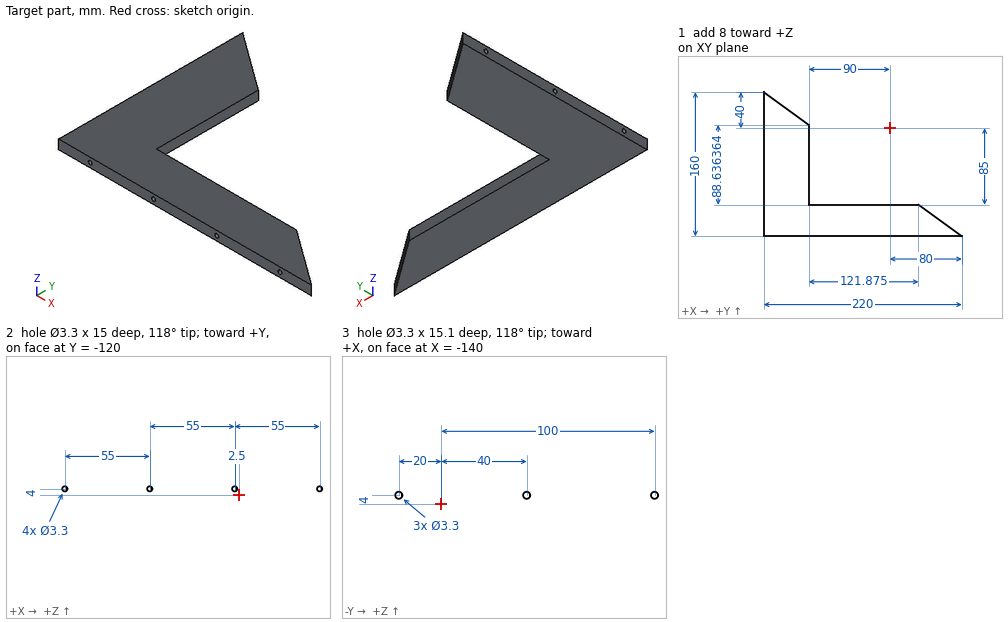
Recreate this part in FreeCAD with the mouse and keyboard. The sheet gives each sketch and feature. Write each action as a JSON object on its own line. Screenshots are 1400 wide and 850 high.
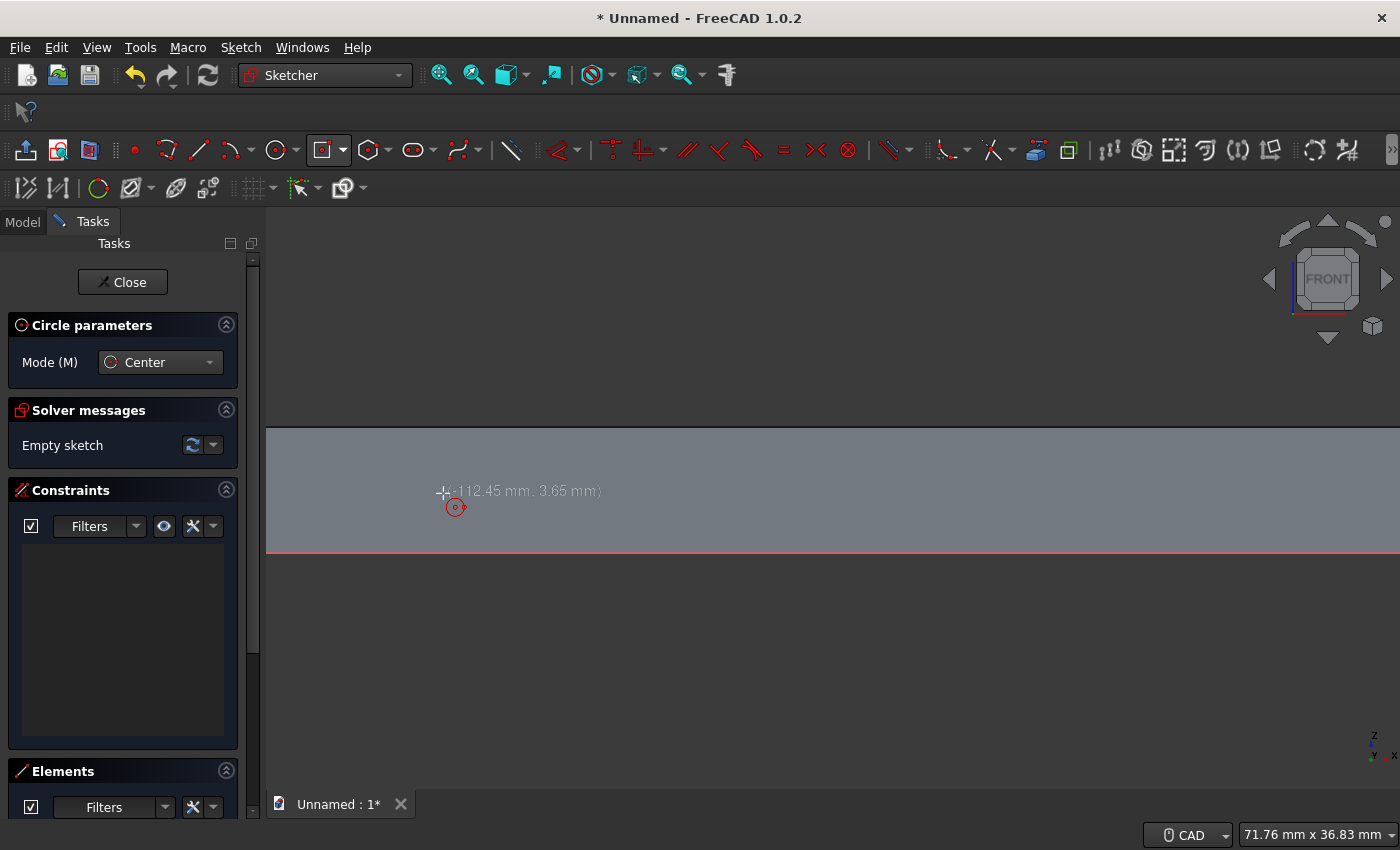
{"action": "scroll", "coordinate": [443, 495], "scroll_direction": "down", "scroll_amount": 7}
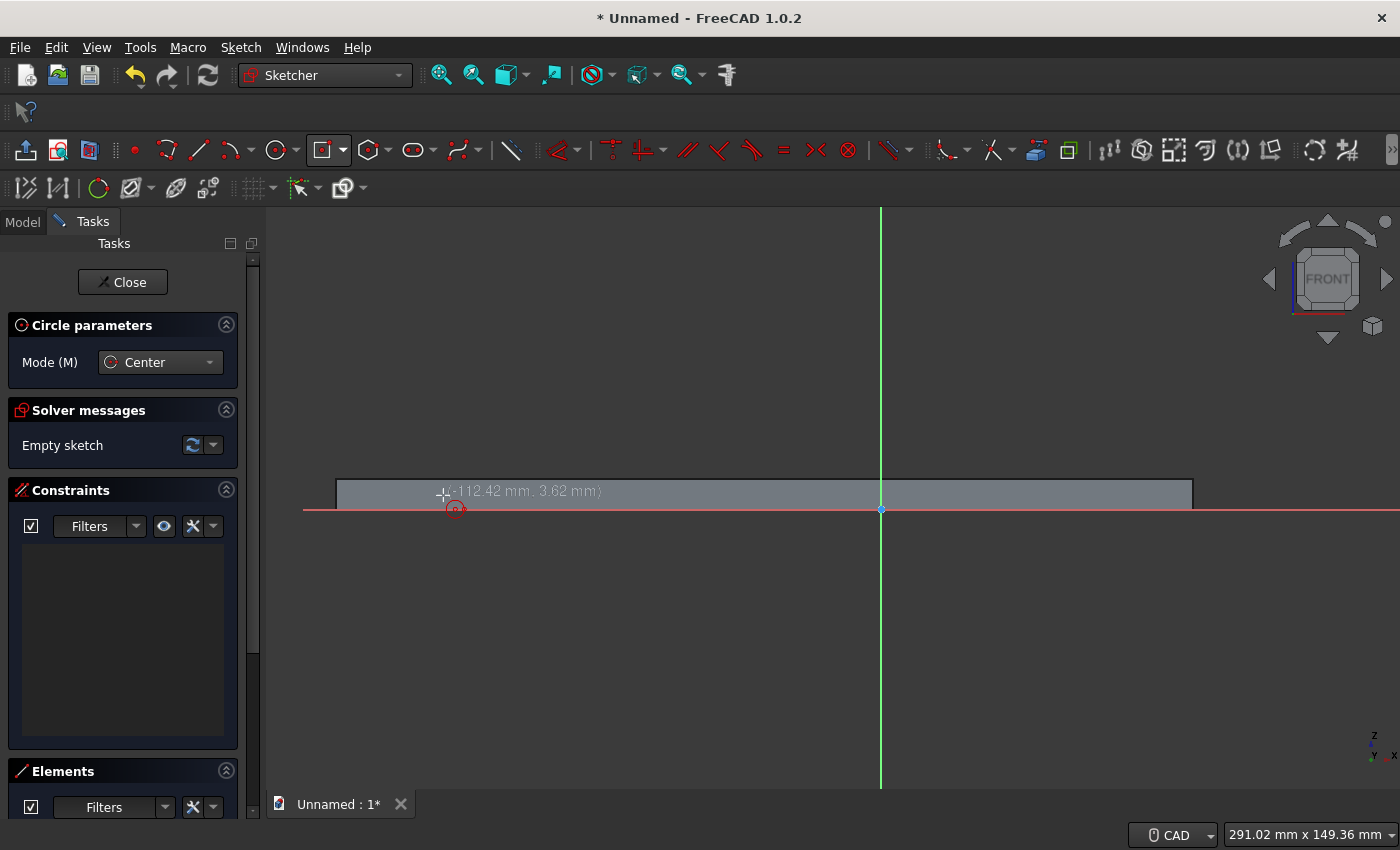
{"action": "left_click", "coordinate": [443, 494]}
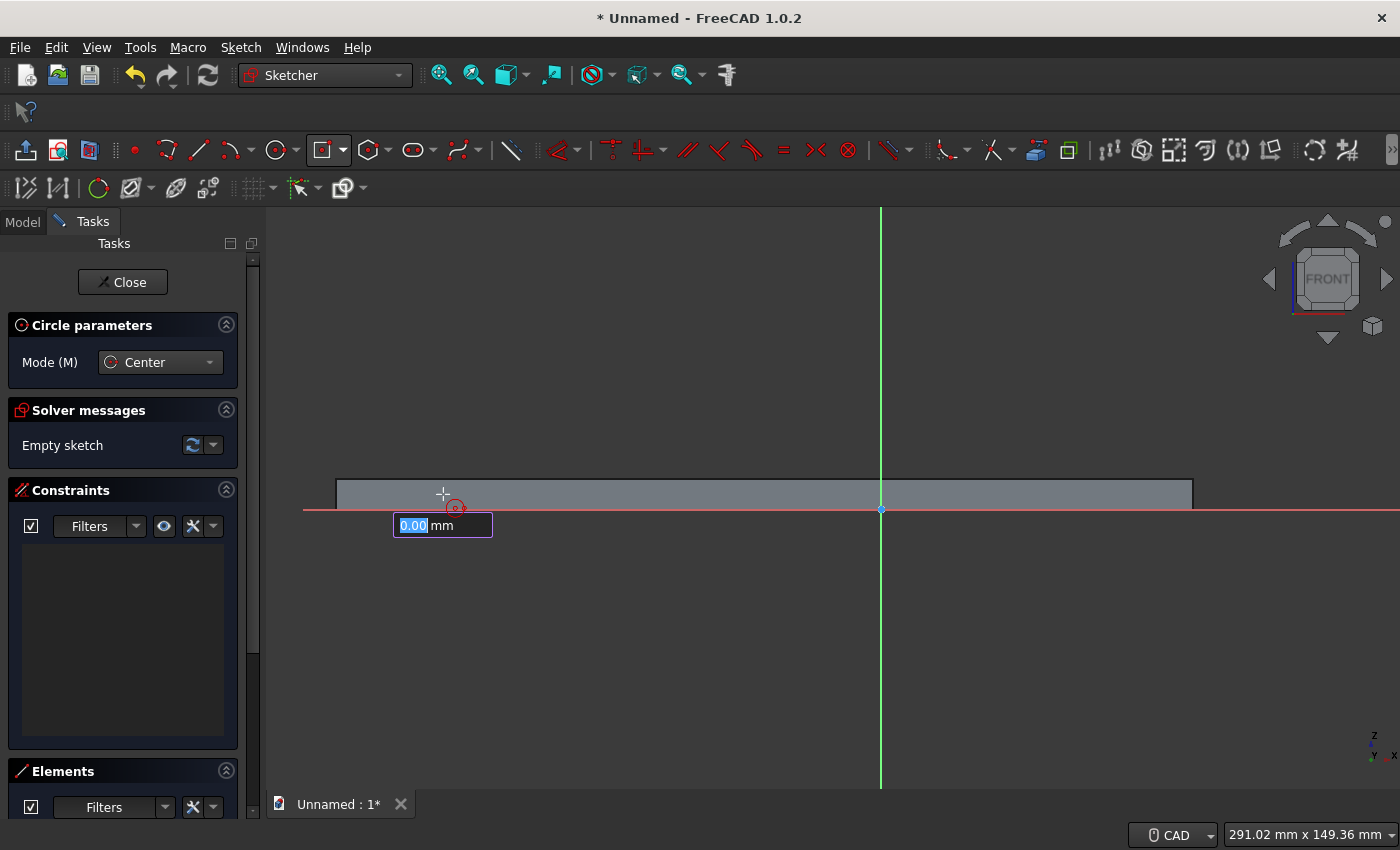
{"action": "scroll", "coordinate": [447, 490], "scroll_direction": "up", "scroll_amount": 5}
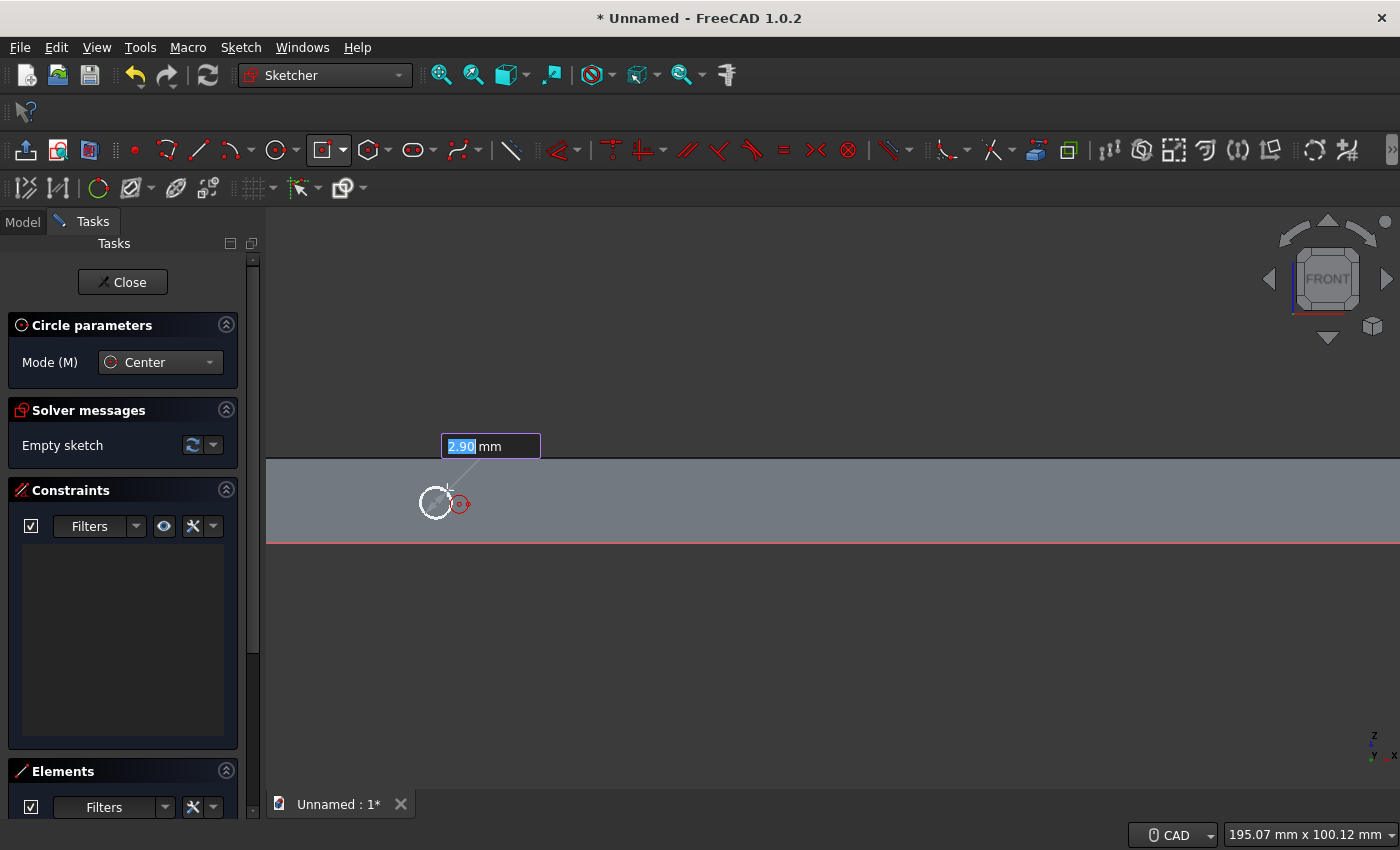
{"action": "left_click", "coordinate": [448, 488]}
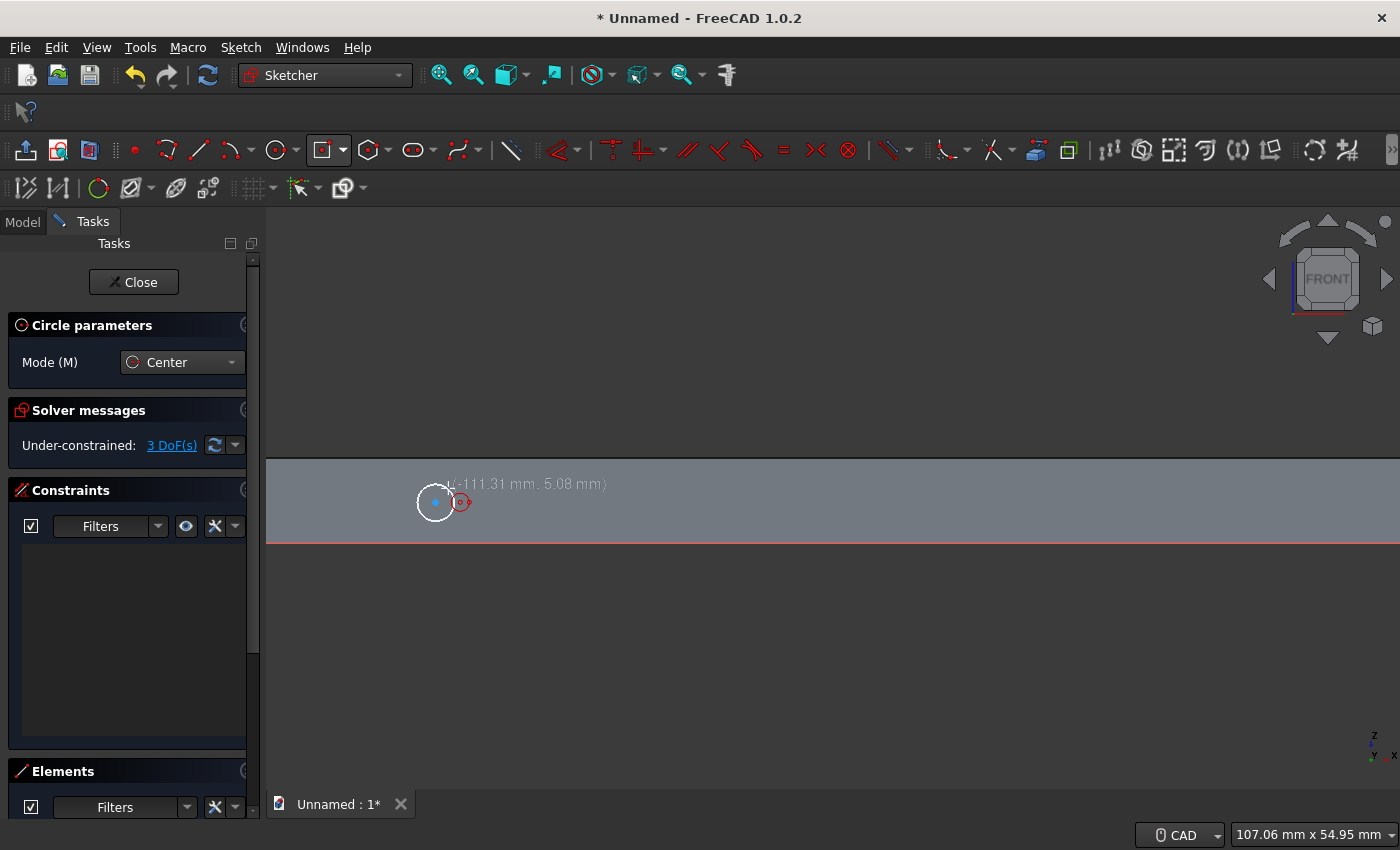
{"action": "scroll", "coordinate": [1018, 500], "scroll_direction": "up", "scroll_amount": 2}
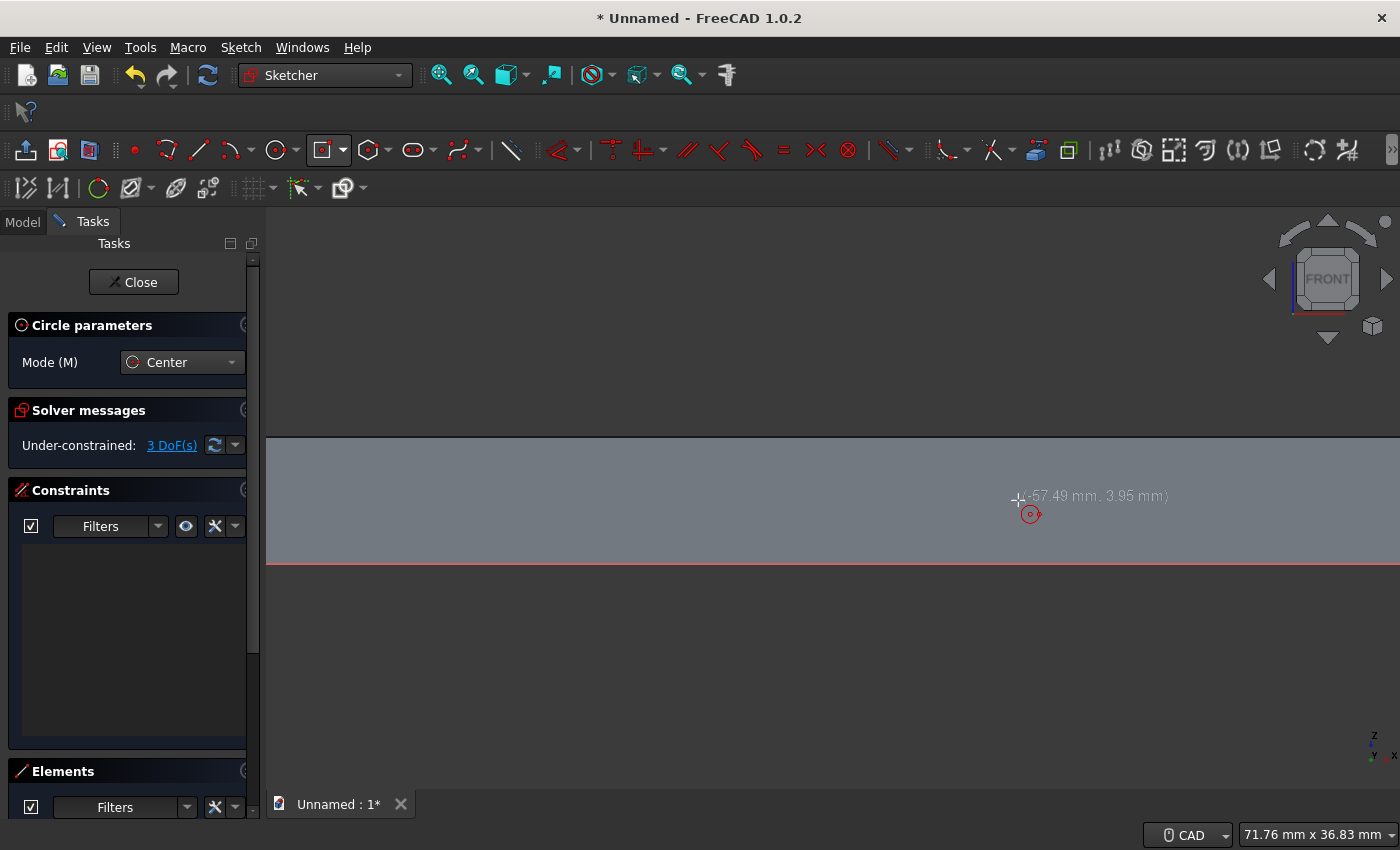
{"action": "scroll", "coordinate": [539, 491], "scroll_direction": "down", "scroll_amount": 7}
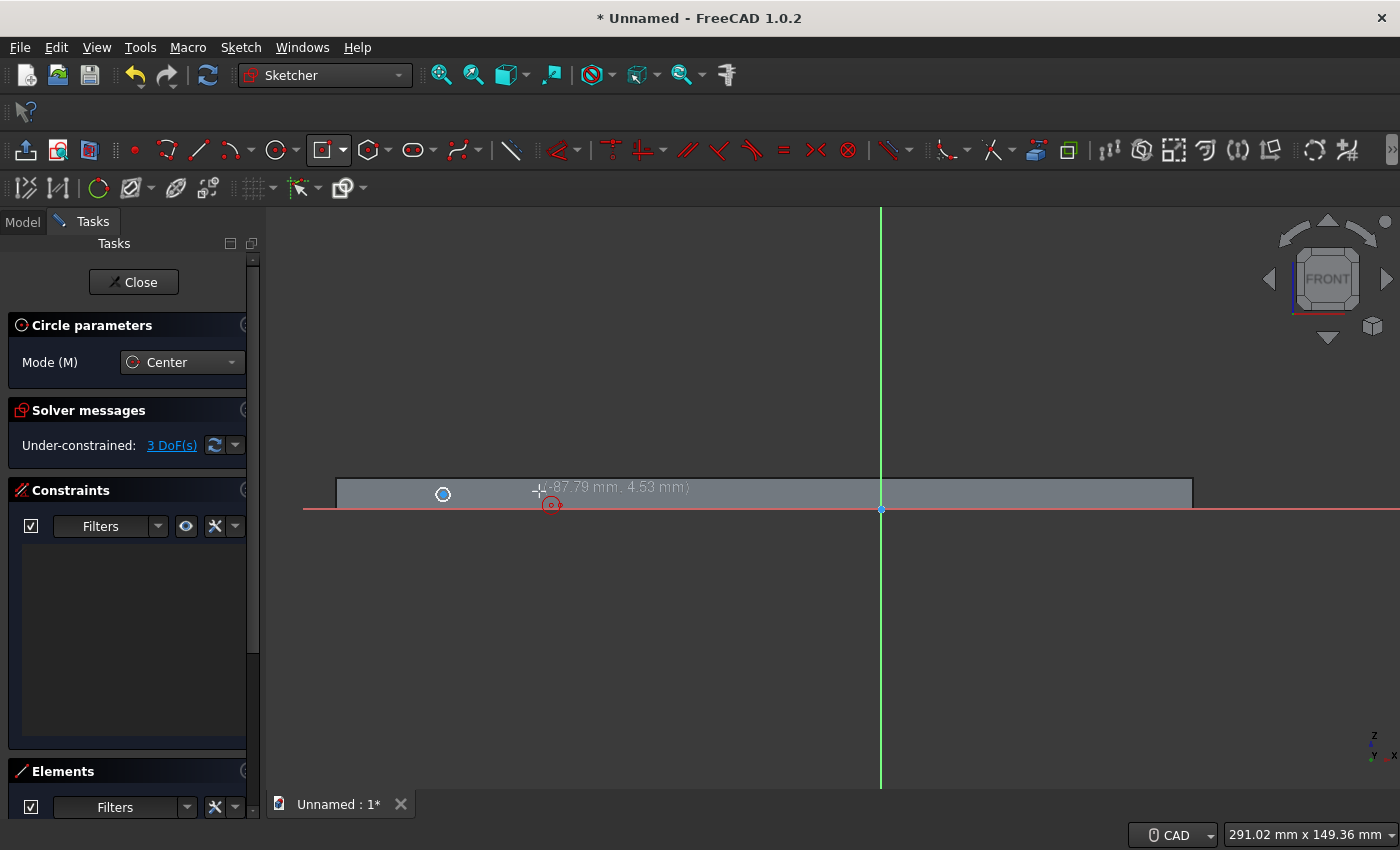
{"action": "left_click", "coordinate": [657, 494]}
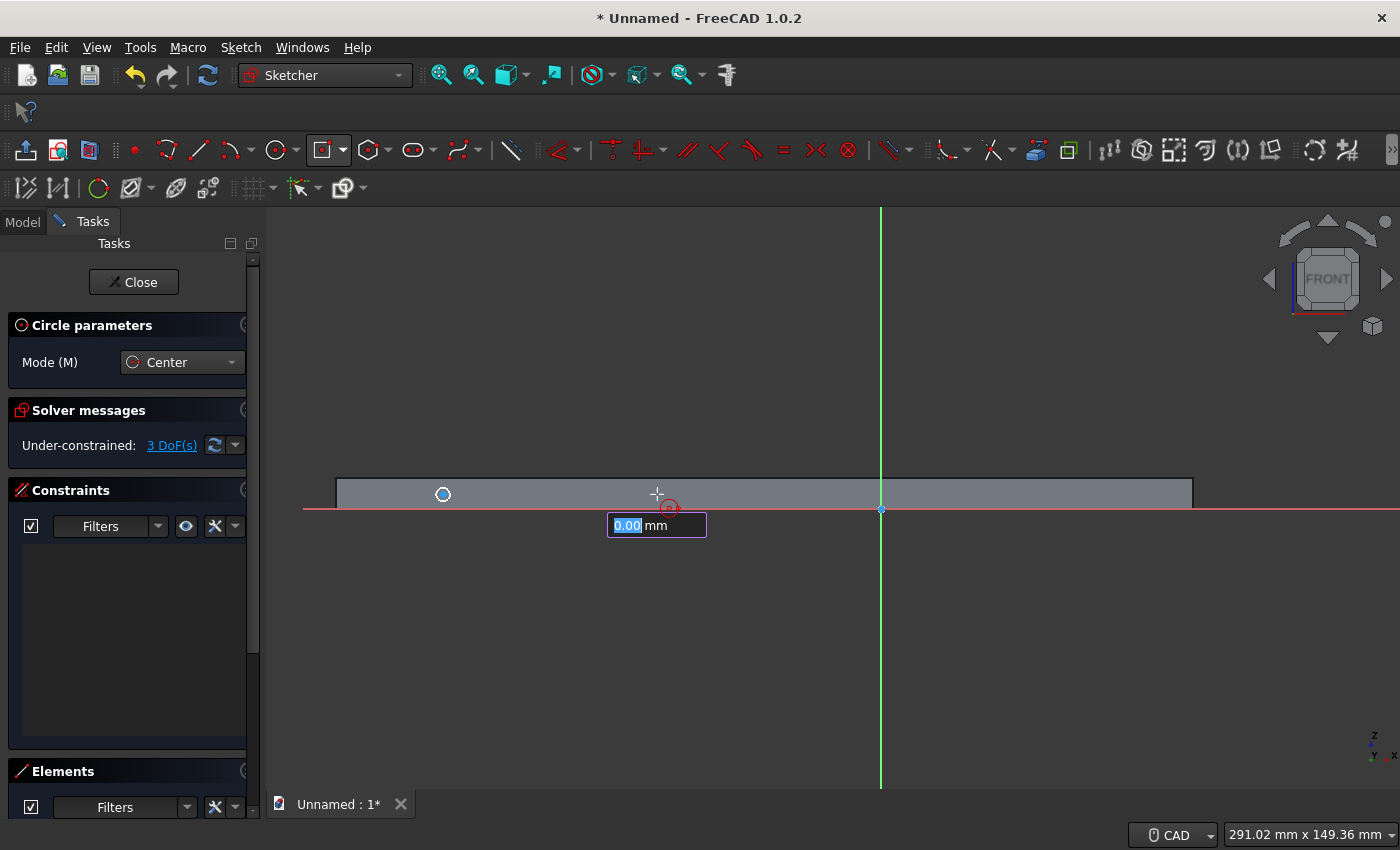
{"action": "scroll", "coordinate": [662, 489], "scroll_direction": "up", "scroll_amount": 5}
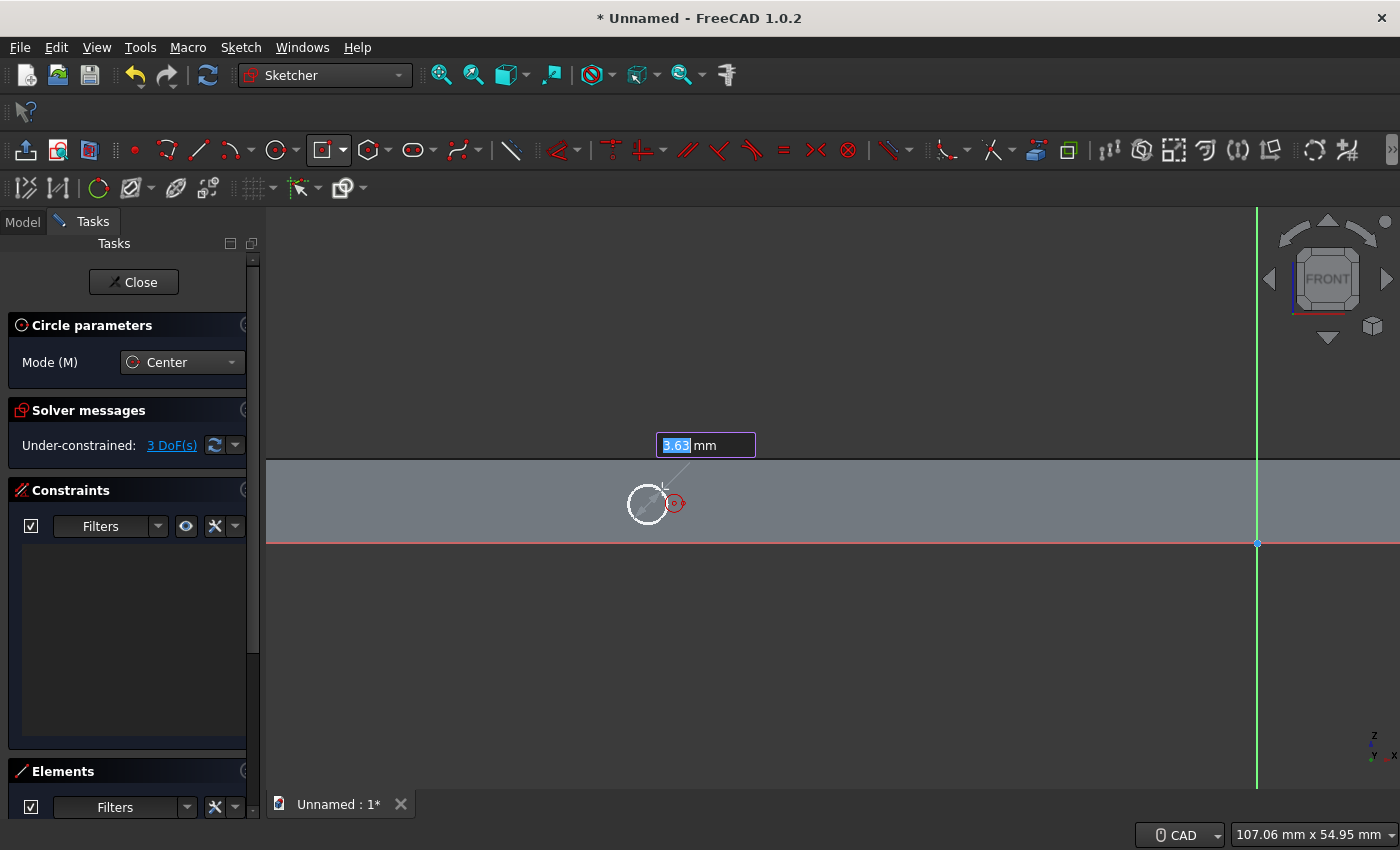
{"action": "left_click", "coordinate": [661, 489]}